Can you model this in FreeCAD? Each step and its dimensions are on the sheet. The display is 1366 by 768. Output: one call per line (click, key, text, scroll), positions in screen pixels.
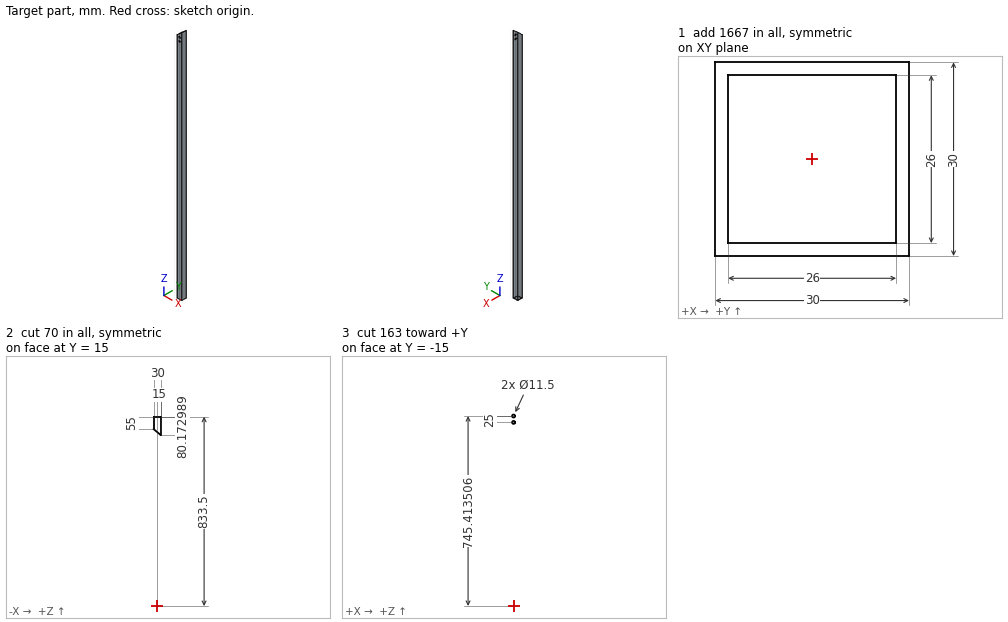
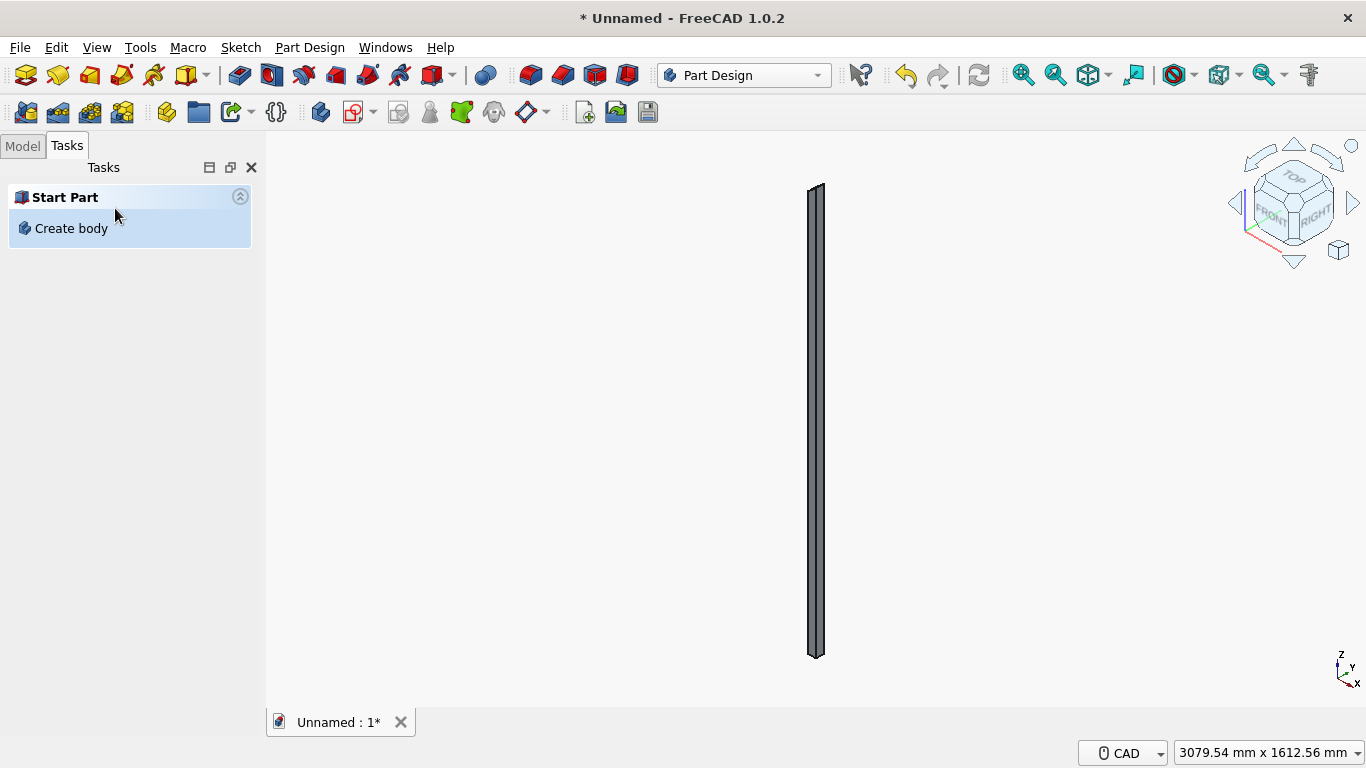
scroll(812, 219, up, 5)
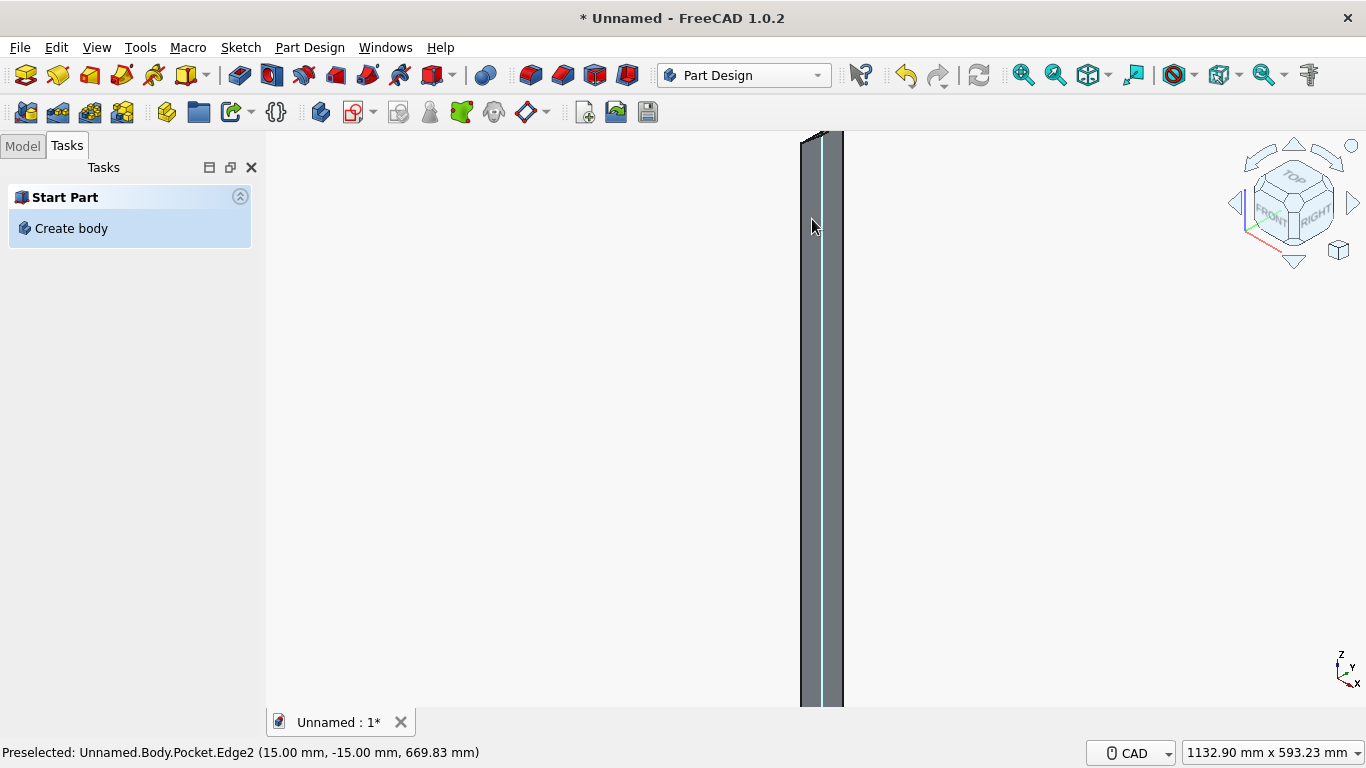
click(812, 220)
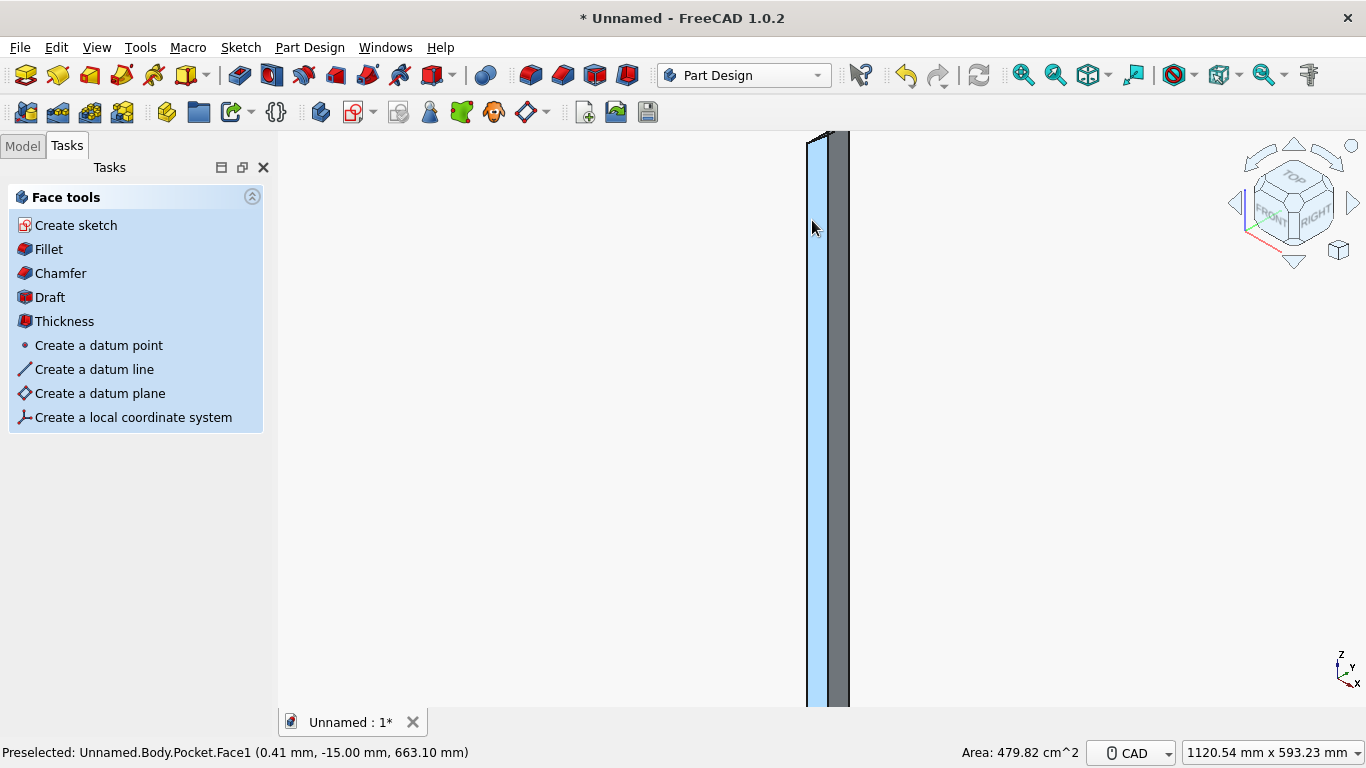
click(354, 112)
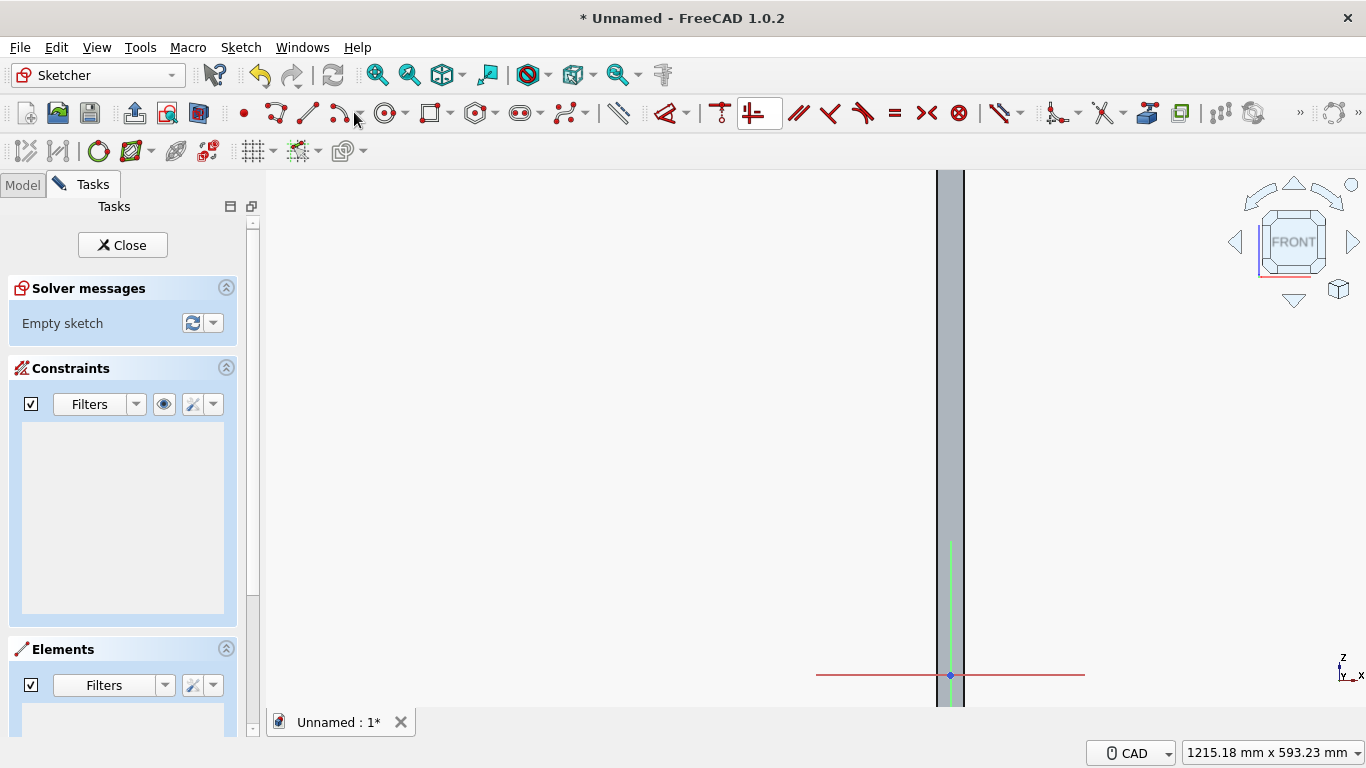
scroll(748, 438, down, 5)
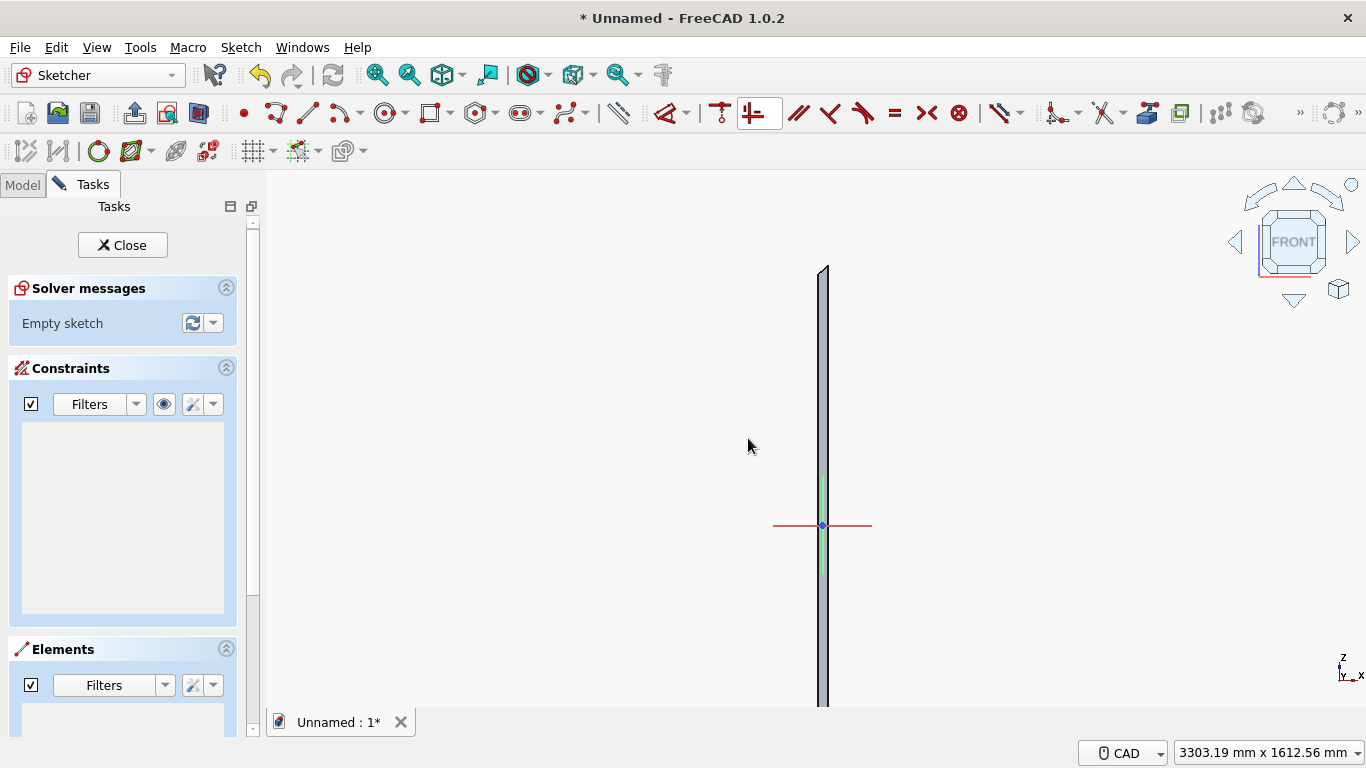
scroll(827, 273, up, 15)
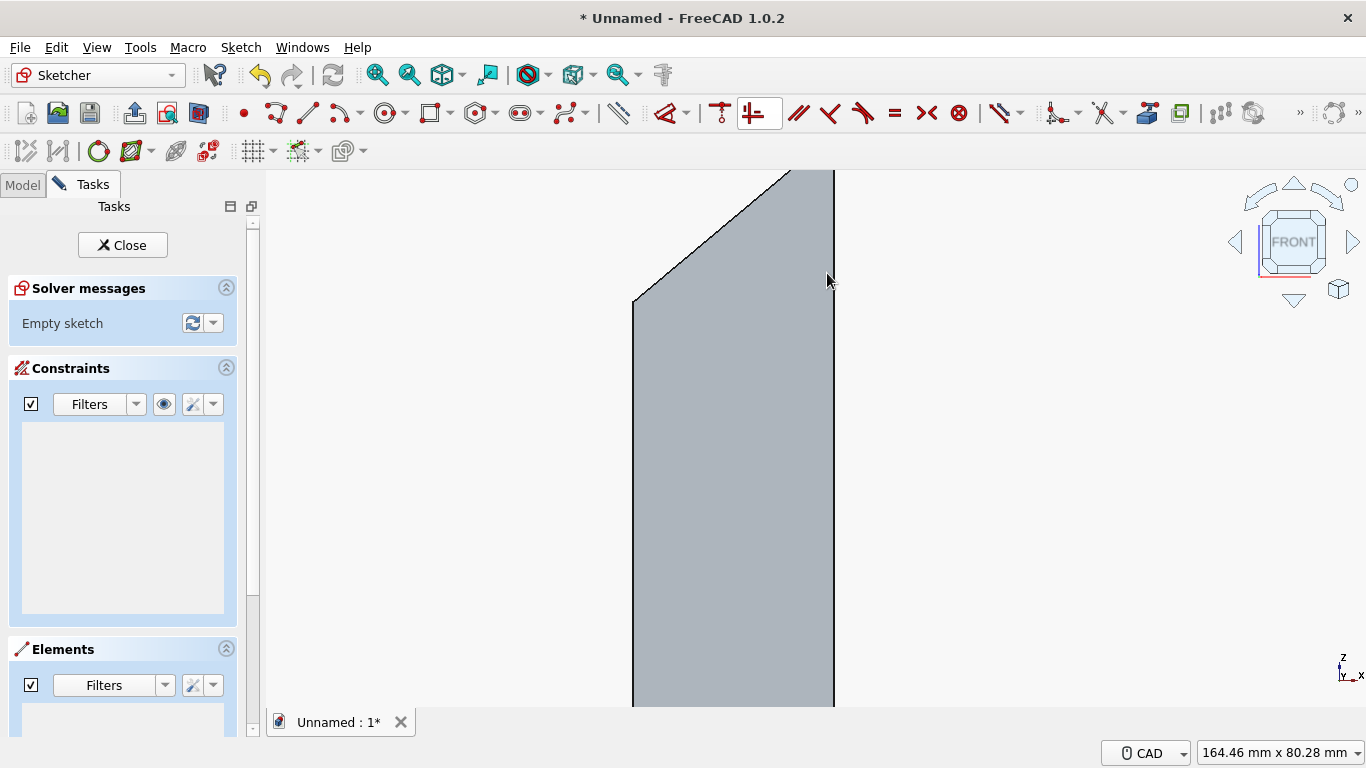
scroll(705, 439, up, 2)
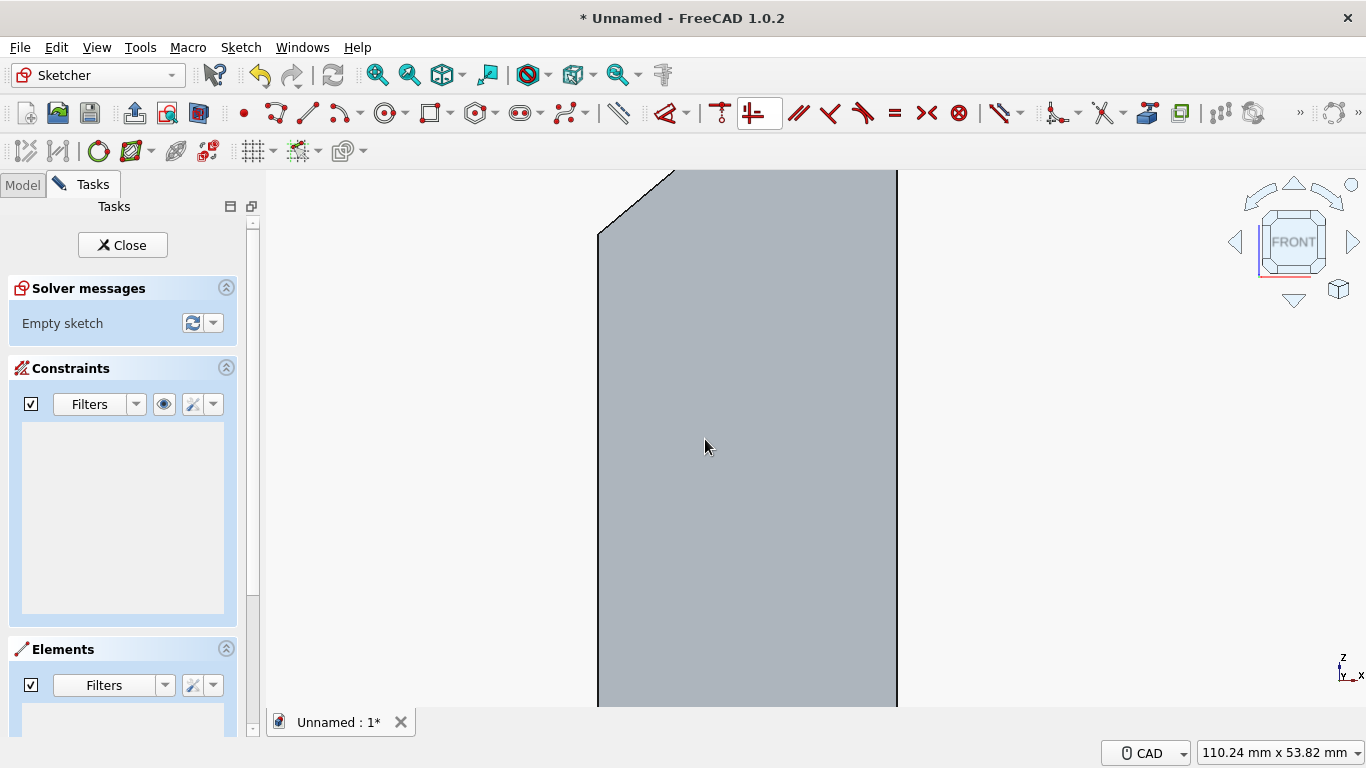
click(386, 114)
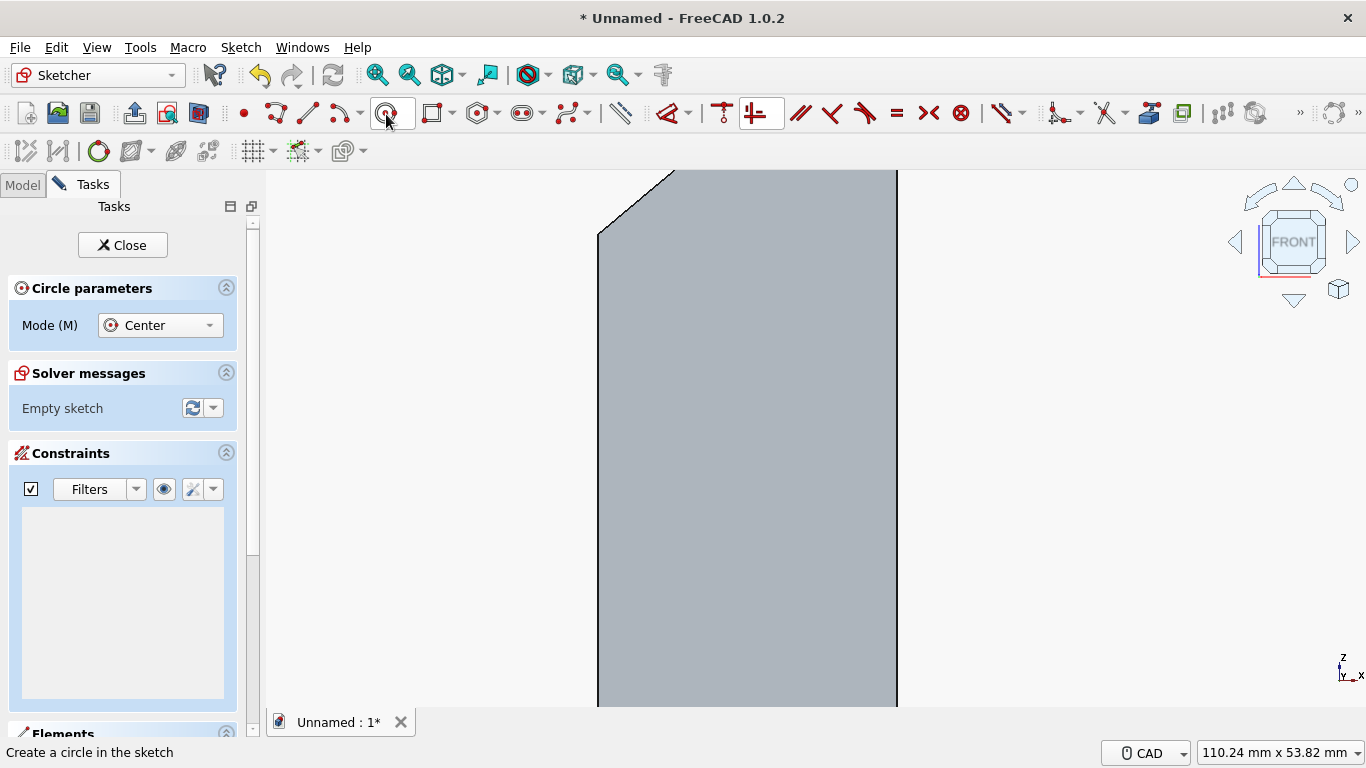
click(747, 314)
click(788, 273)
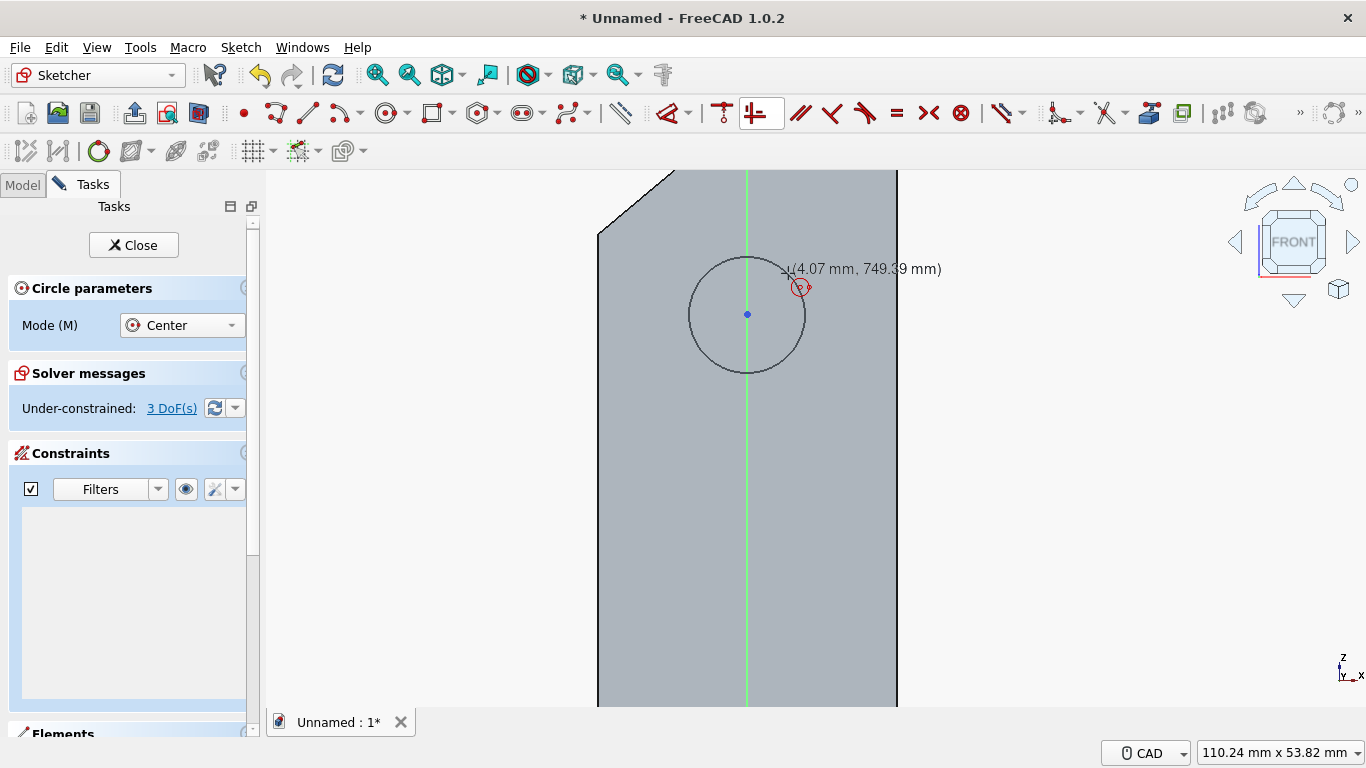
click(747, 563)
click(788, 523)
key(Escape)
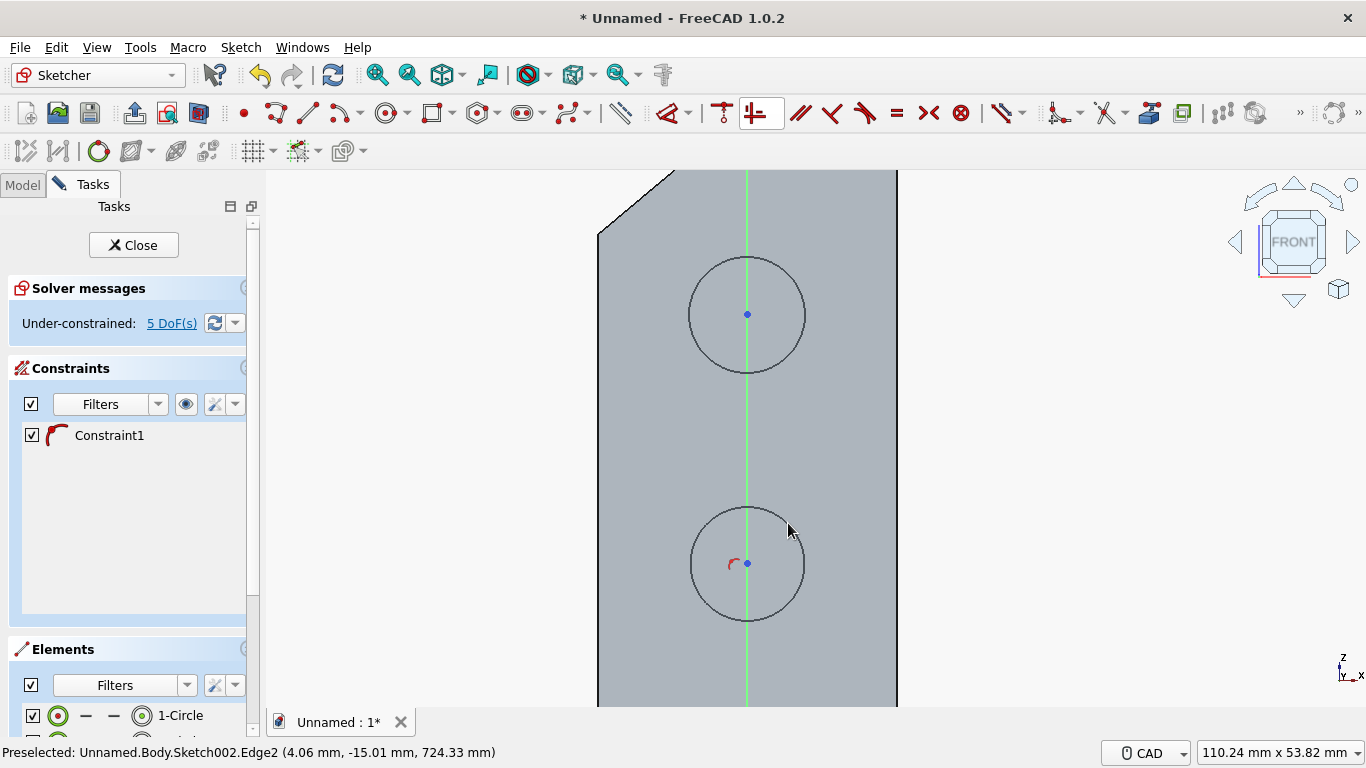
click(788, 274)